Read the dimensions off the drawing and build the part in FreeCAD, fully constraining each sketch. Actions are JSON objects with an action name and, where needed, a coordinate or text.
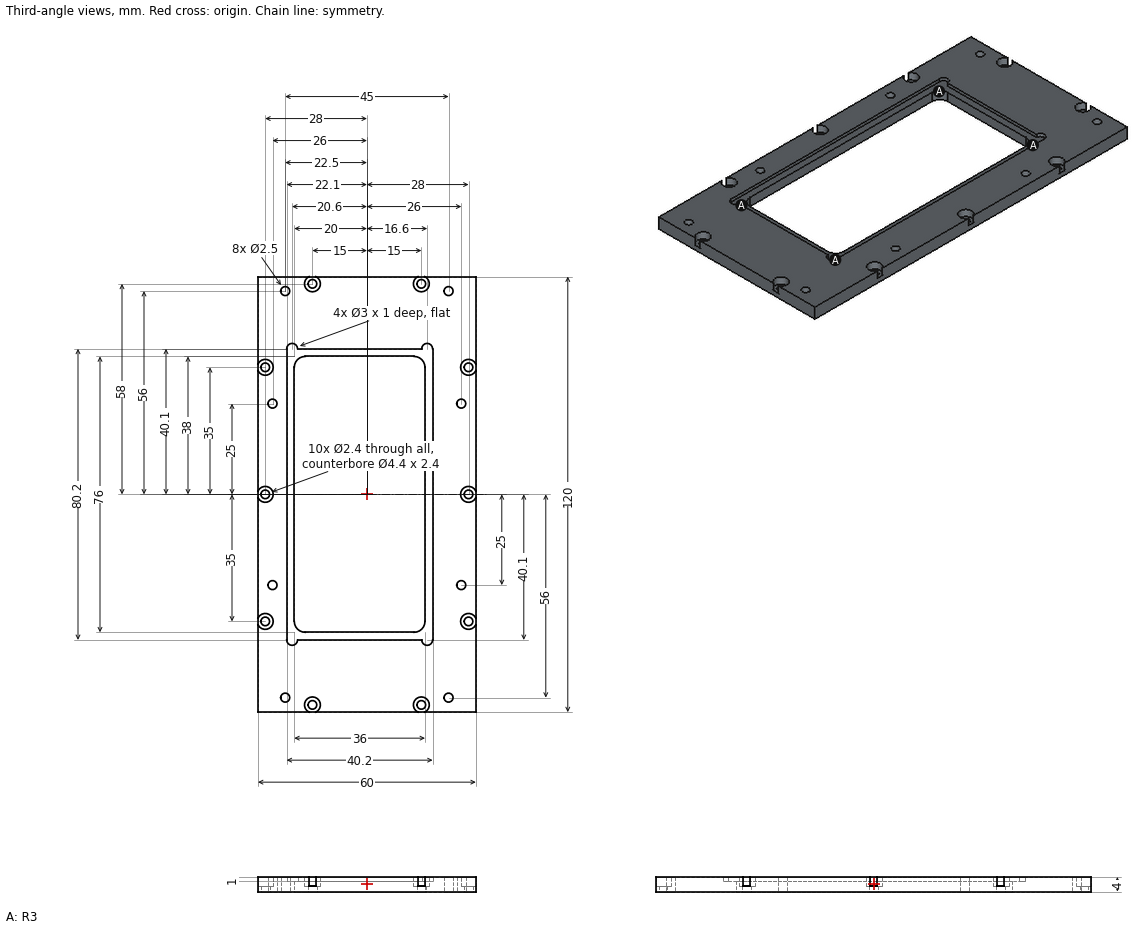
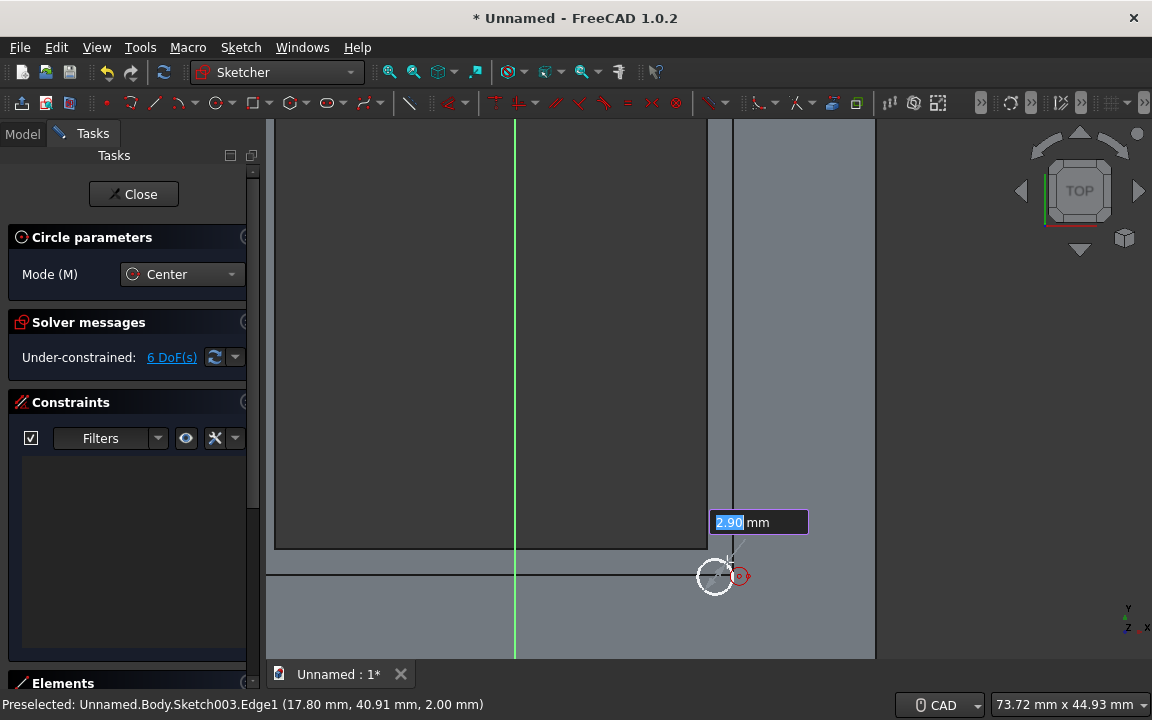
{"action": "left_click", "coordinate": [727, 562]}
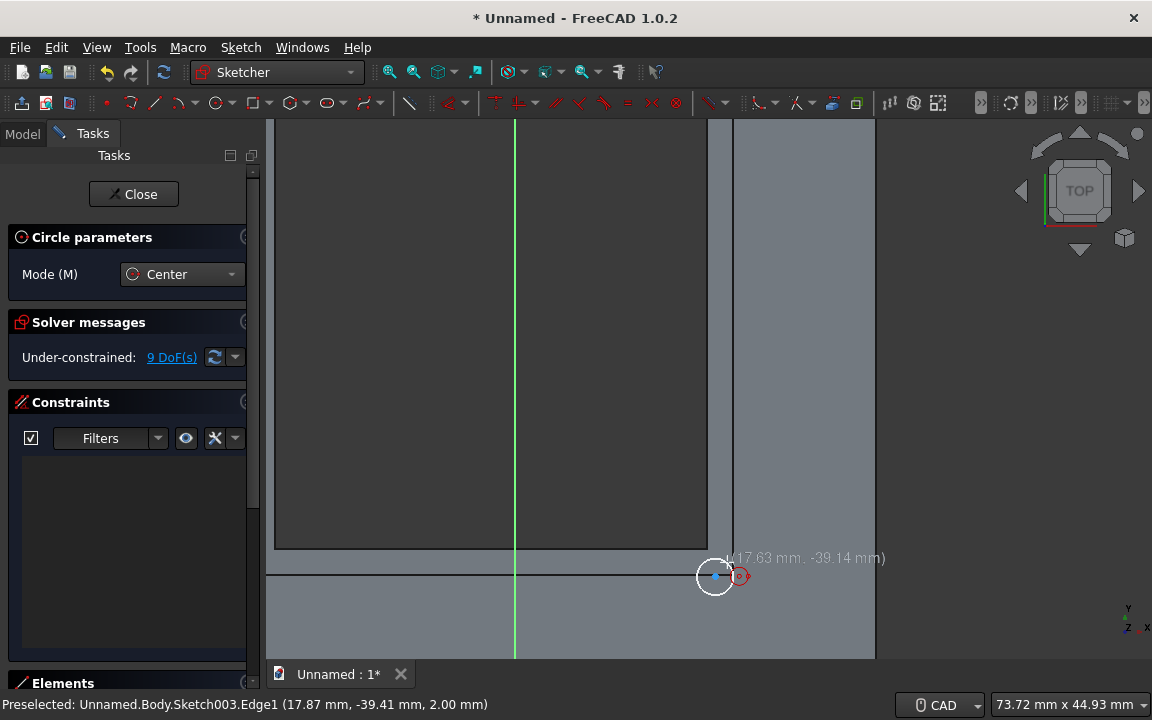
{"action": "scroll", "coordinate": [727, 561], "scroll_direction": "down", "scroll_amount": 5}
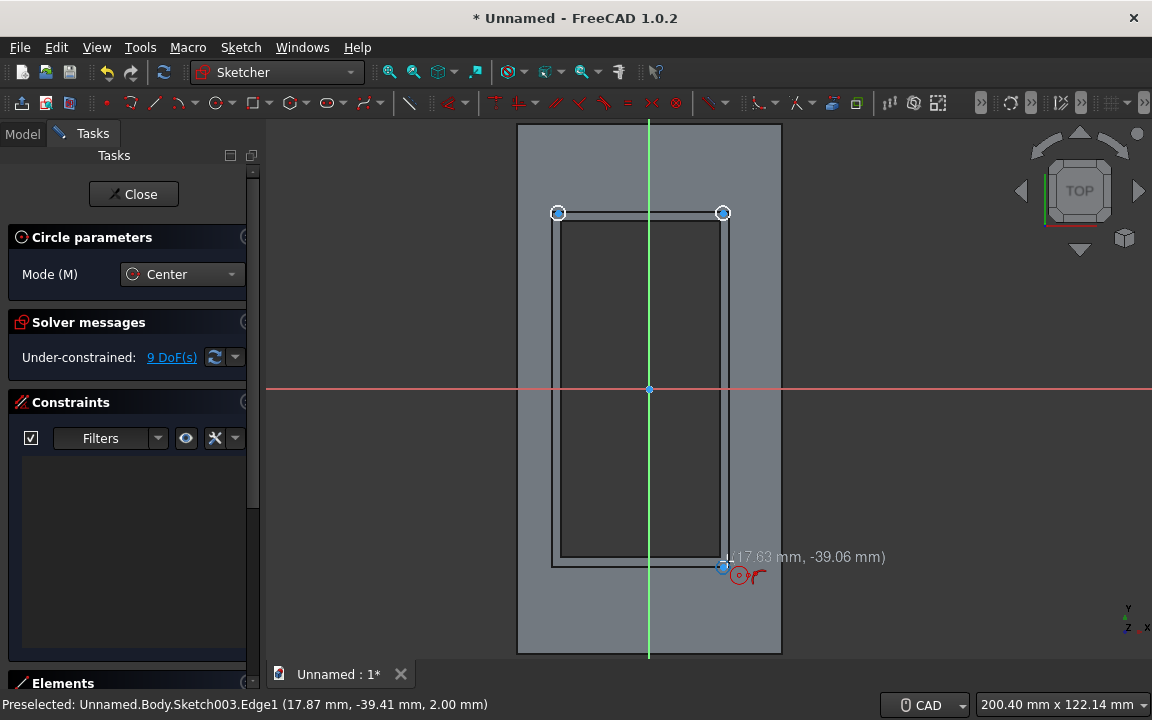
{"action": "scroll", "coordinate": [558, 566], "scroll_direction": "up", "scroll_amount": 7}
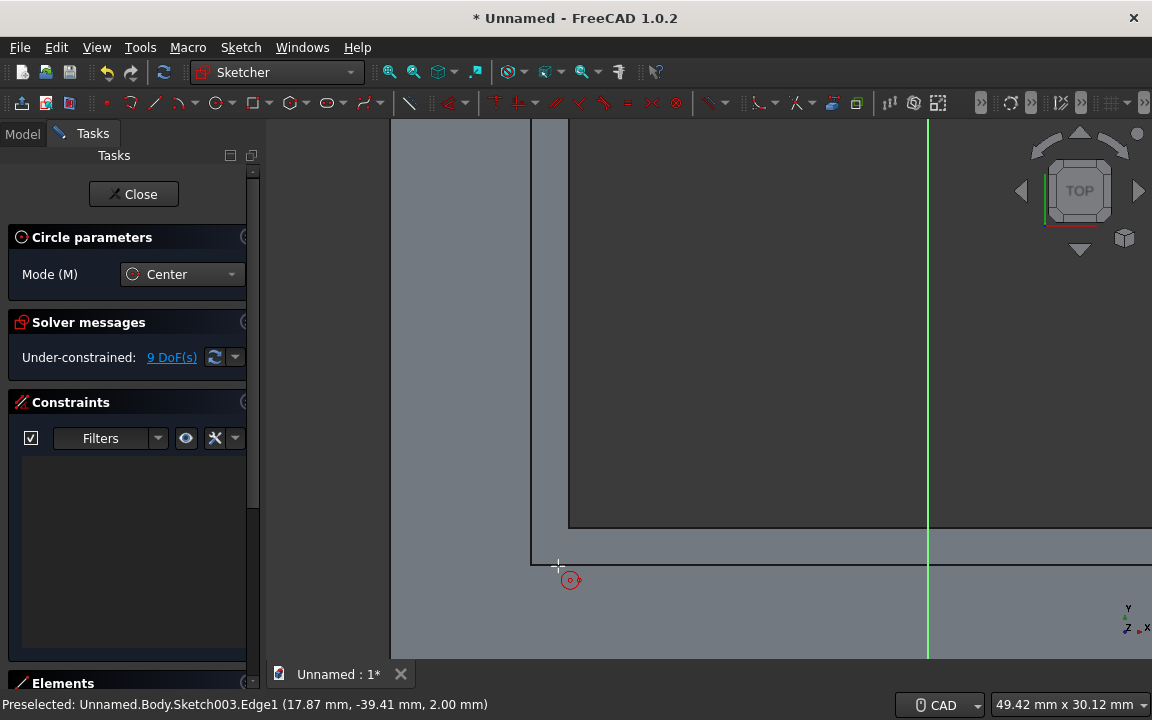
{"action": "scroll", "coordinate": [558, 567], "scroll_direction": "down", "scroll_amount": 7}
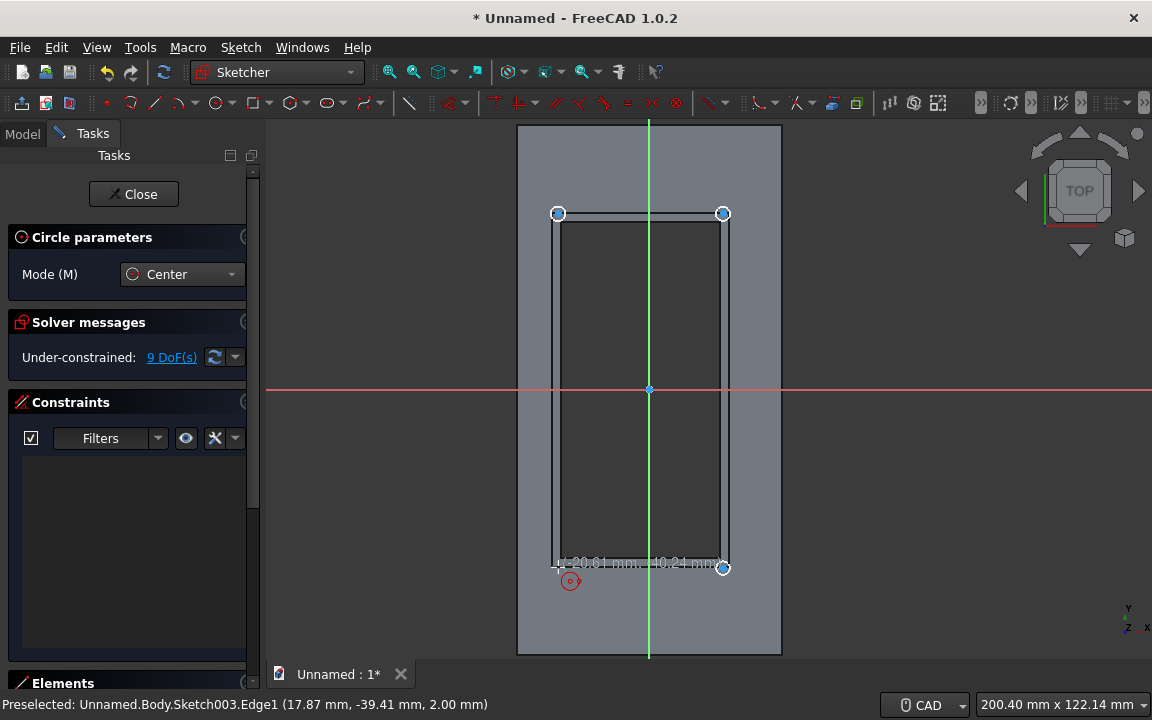
{"action": "left_click", "coordinate": [558, 567]}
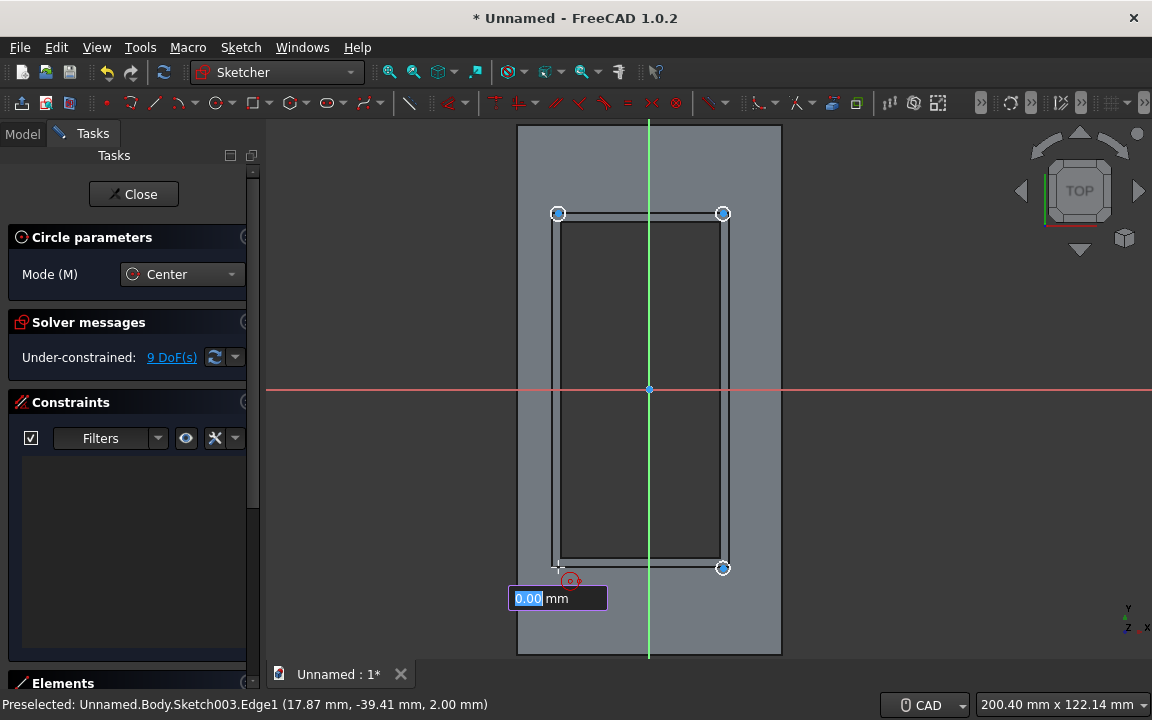
{"action": "scroll", "coordinate": [563, 563], "scroll_direction": "up", "scroll_amount": 5}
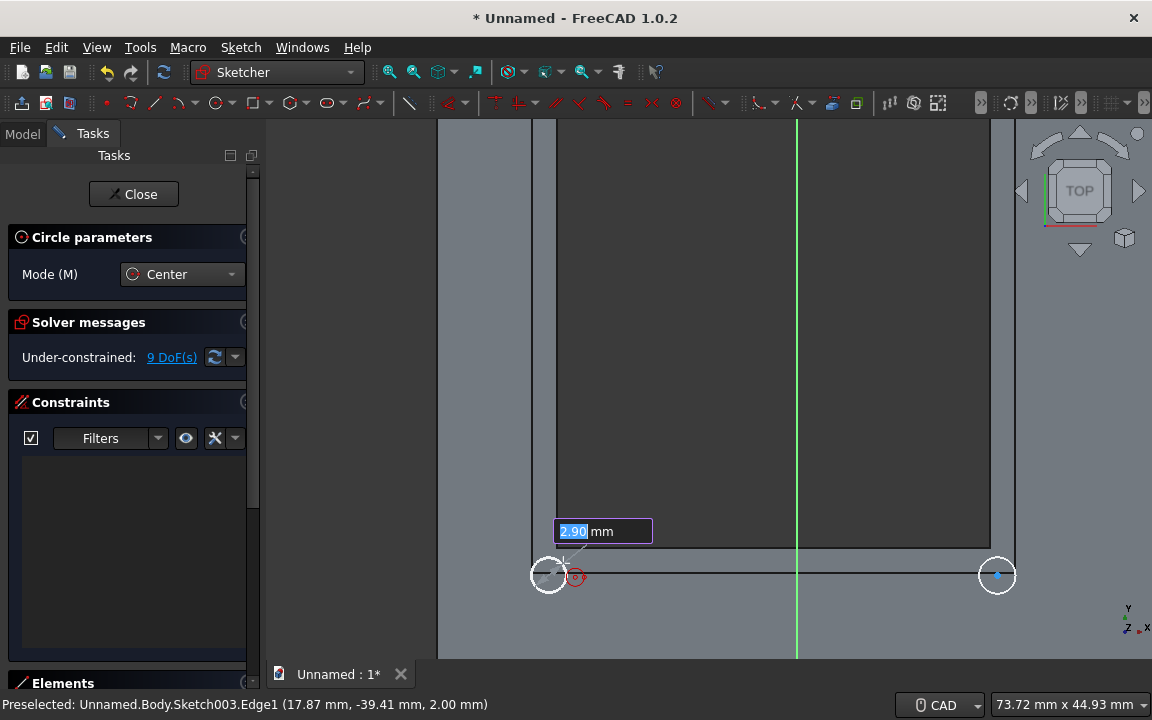
{"action": "left_click", "coordinate": [562, 560]}
{"action": "key", "text": "Escape"}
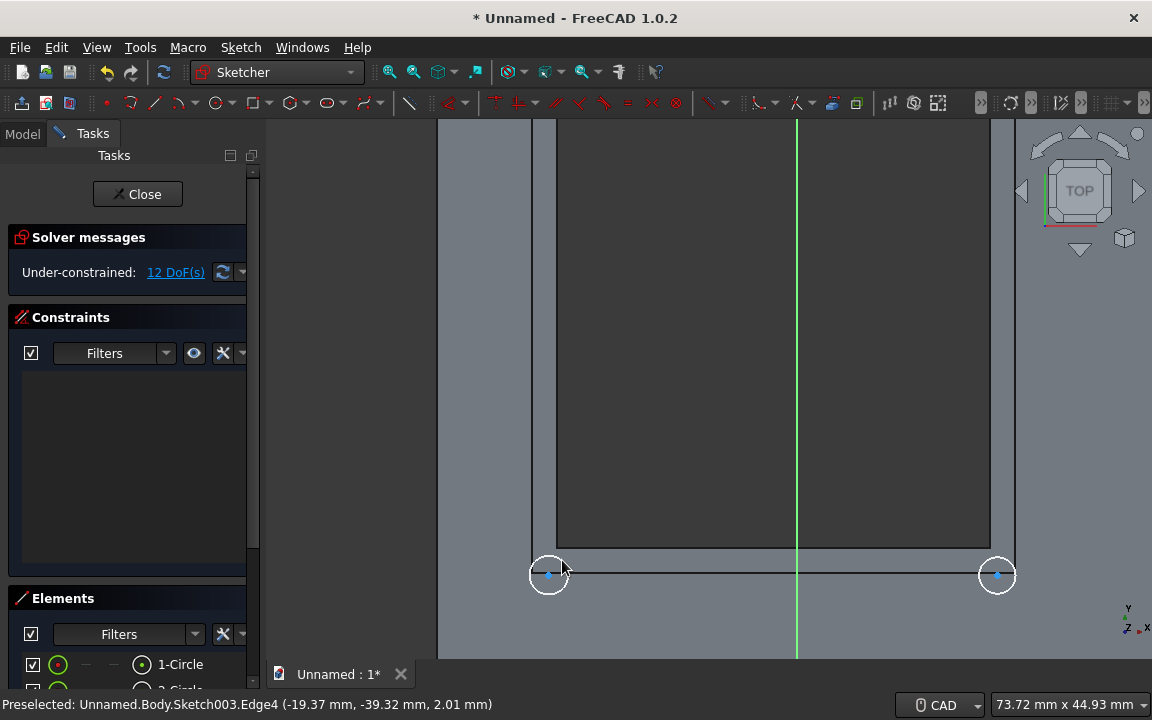
{"action": "scroll", "coordinate": [563, 562], "scroll_direction": "down", "scroll_amount": 5}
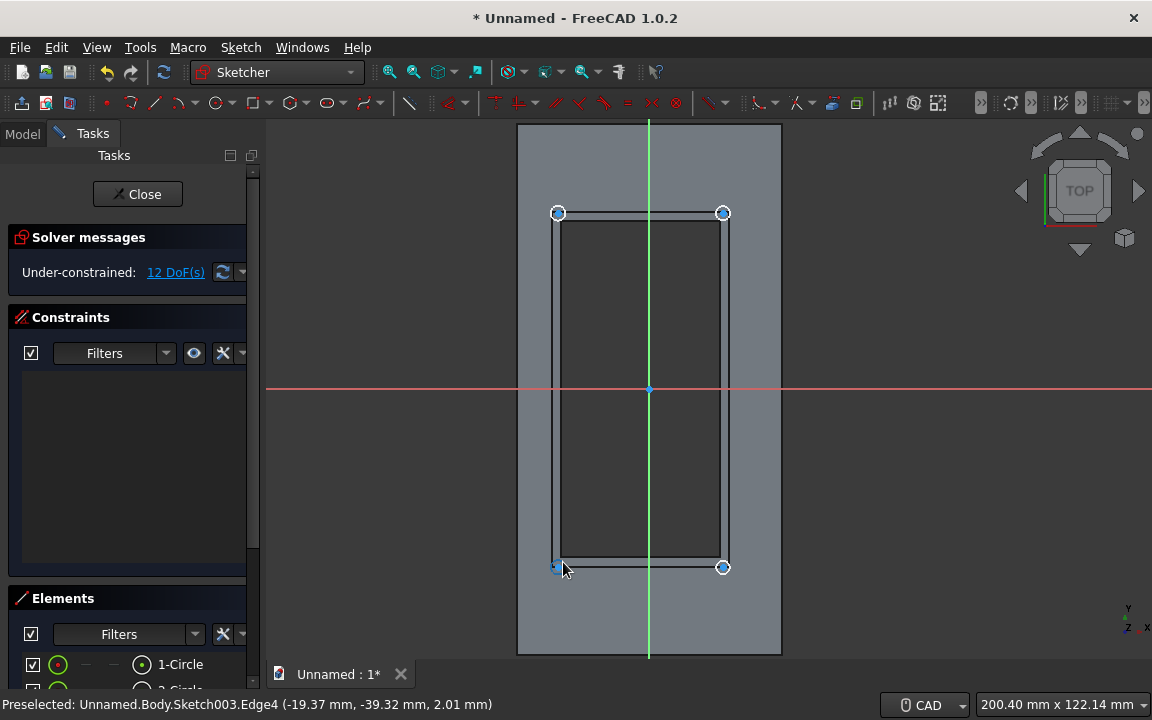
{"action": "scroll", "coordinate": [563, 208], "scroll_direction": "up", "scroll_amount": 4}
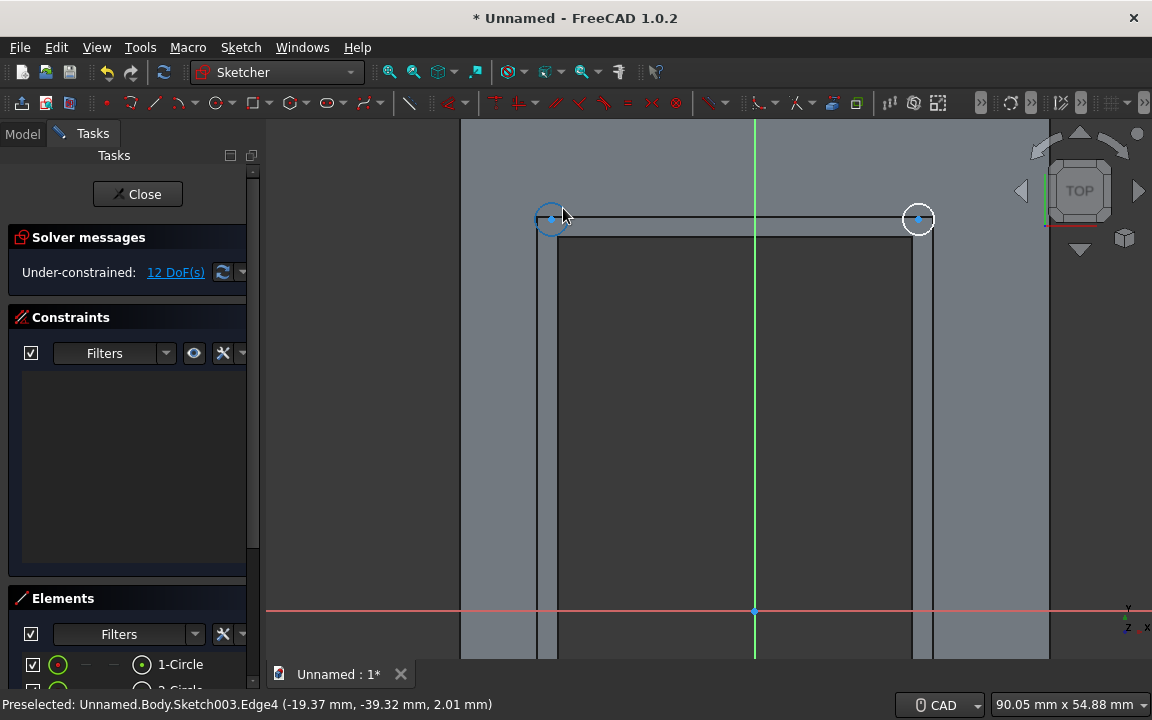
{"action": "left_click", "coordinate": [563, 208]}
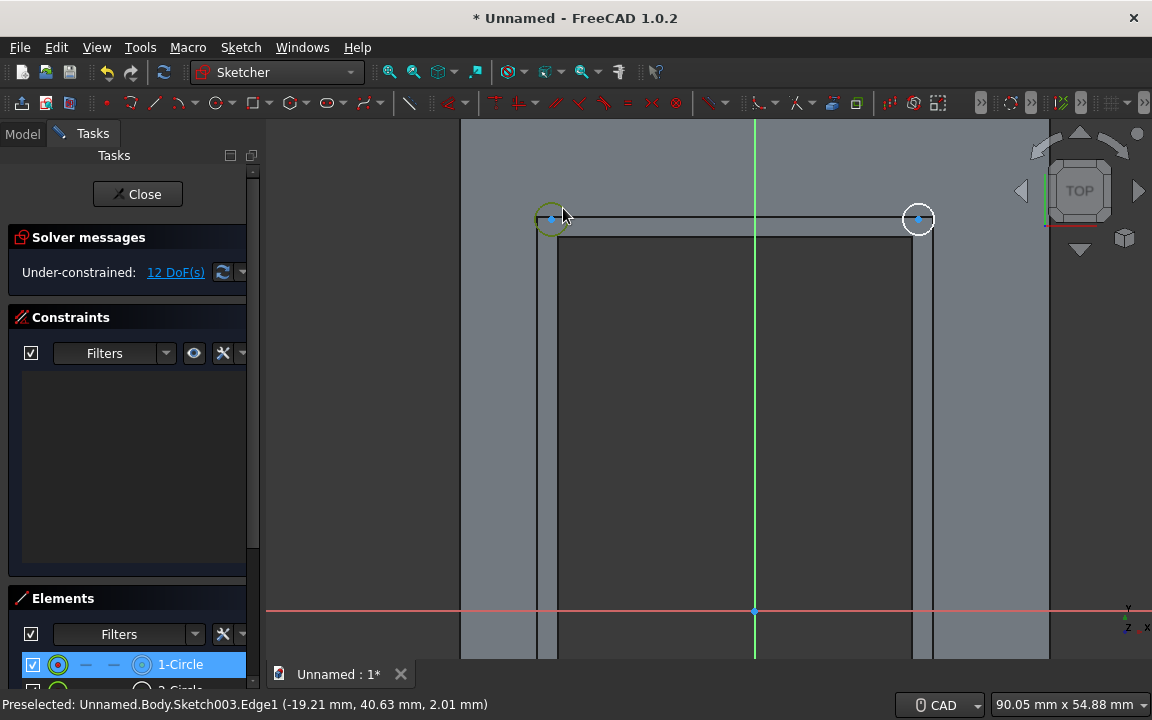
{"action": "left_click", "coordinate": [930, 208]}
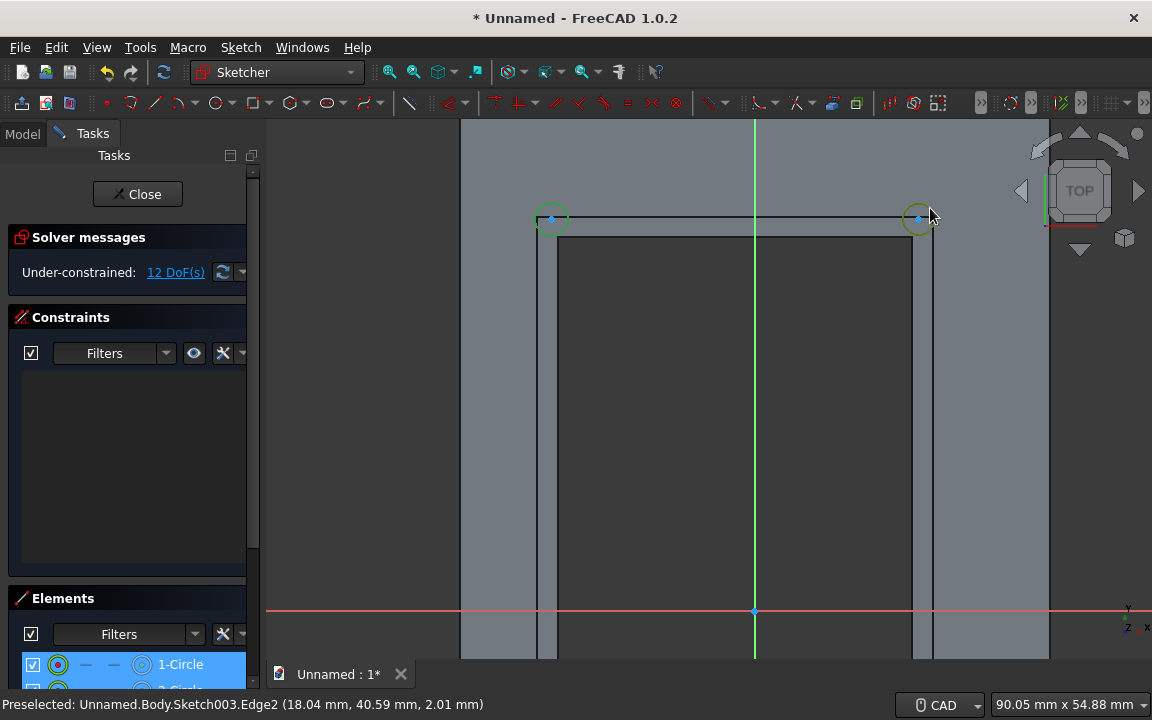
{"action": "scroll", "coordinate": [563, 208], "scroll_direction": "down", "scroll_amount": 4}